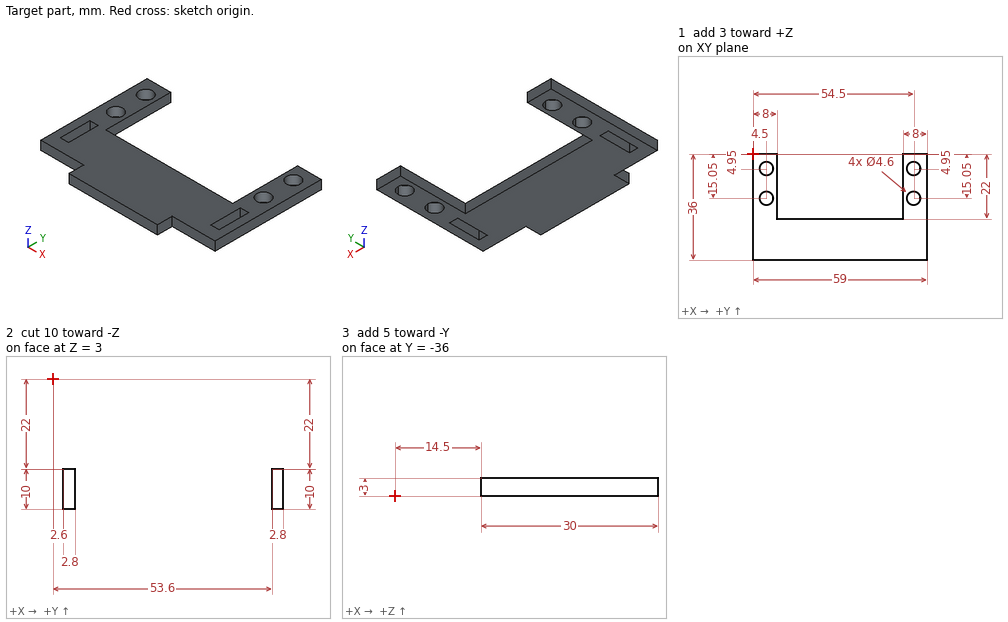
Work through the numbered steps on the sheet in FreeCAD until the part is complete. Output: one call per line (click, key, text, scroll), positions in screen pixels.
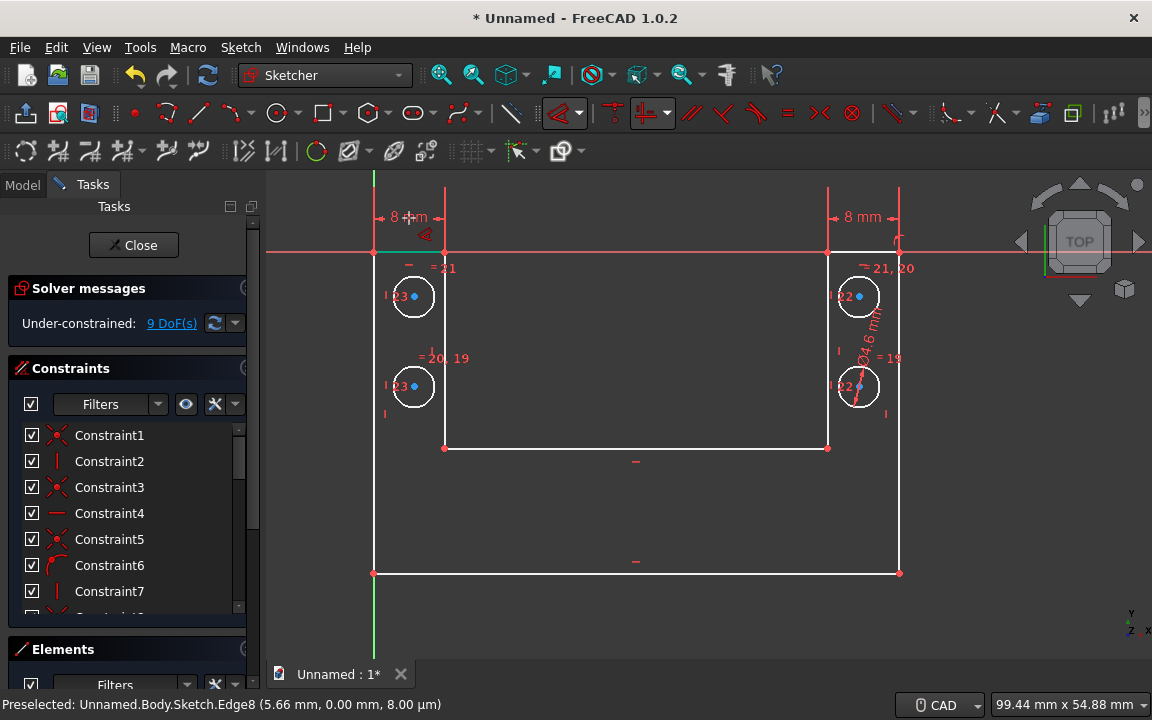
click(374, 349)
click(340, 413)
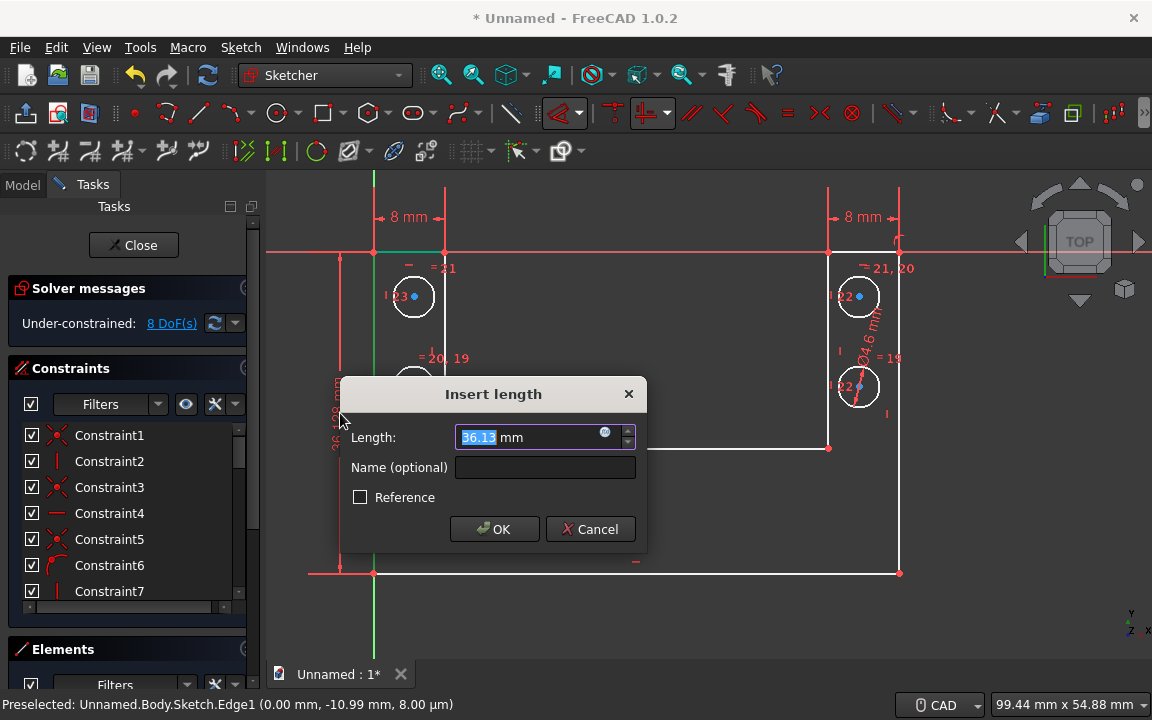
text(36)
key(Return)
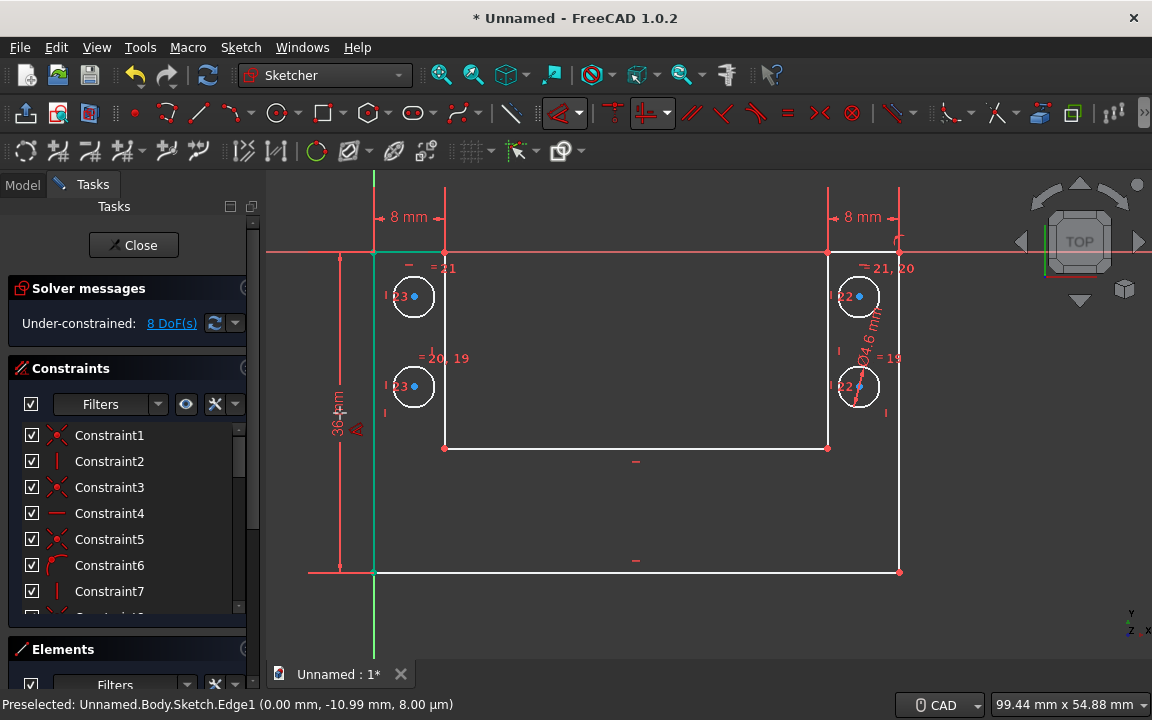
click(531, 573)
click(636, 607)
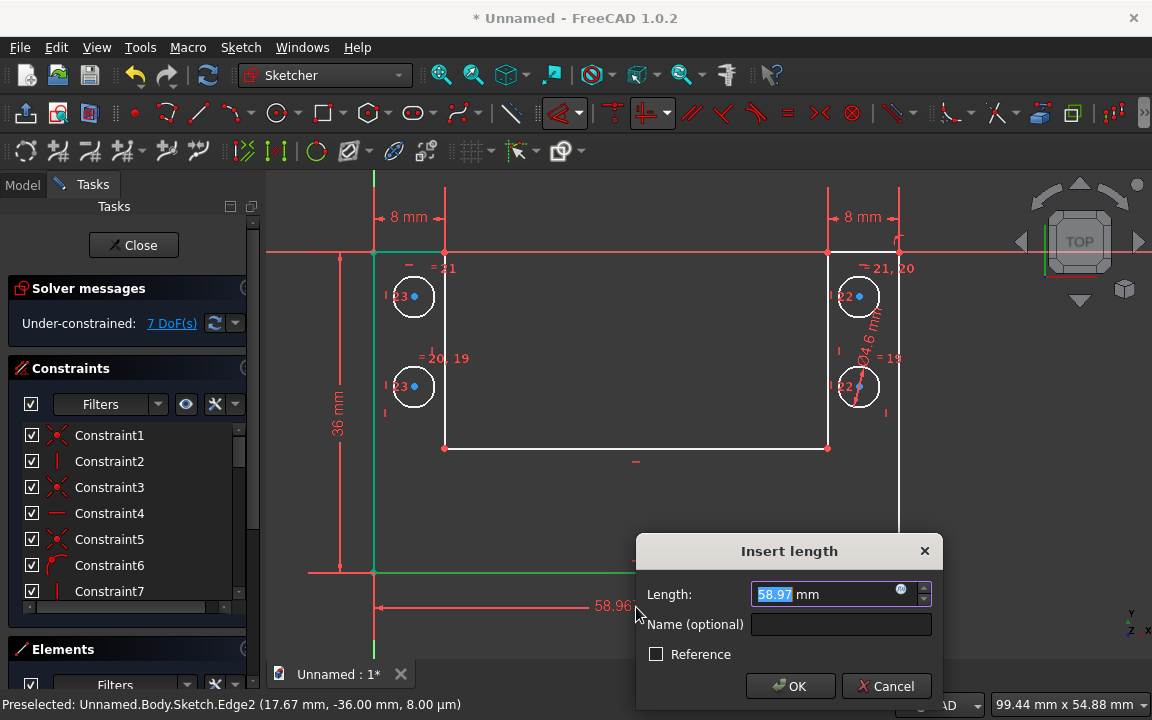
text(59)
key(Return)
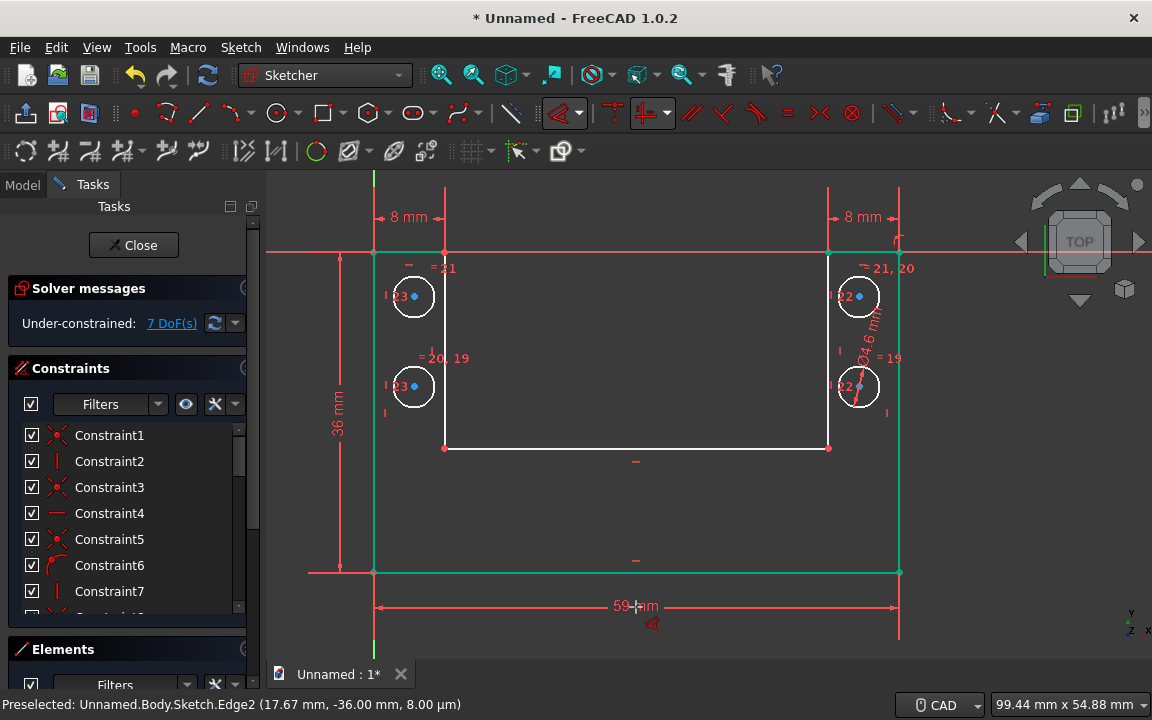
click(828, 311)
click(794, 351)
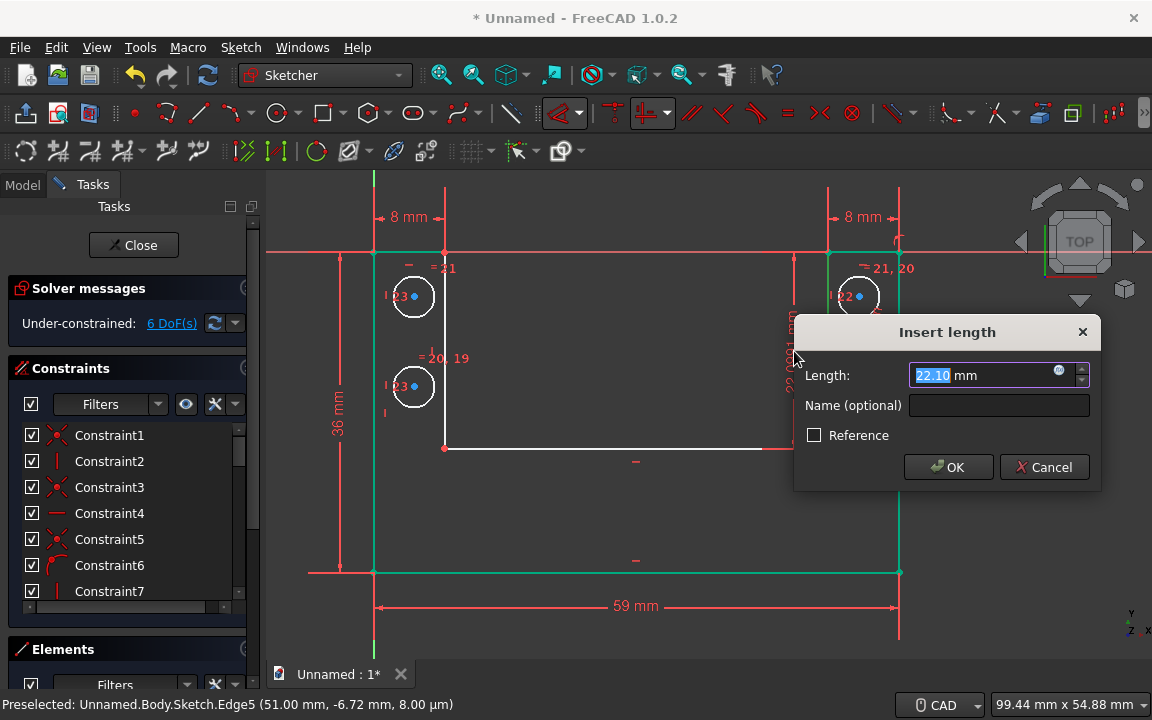
text(22)
key(Return)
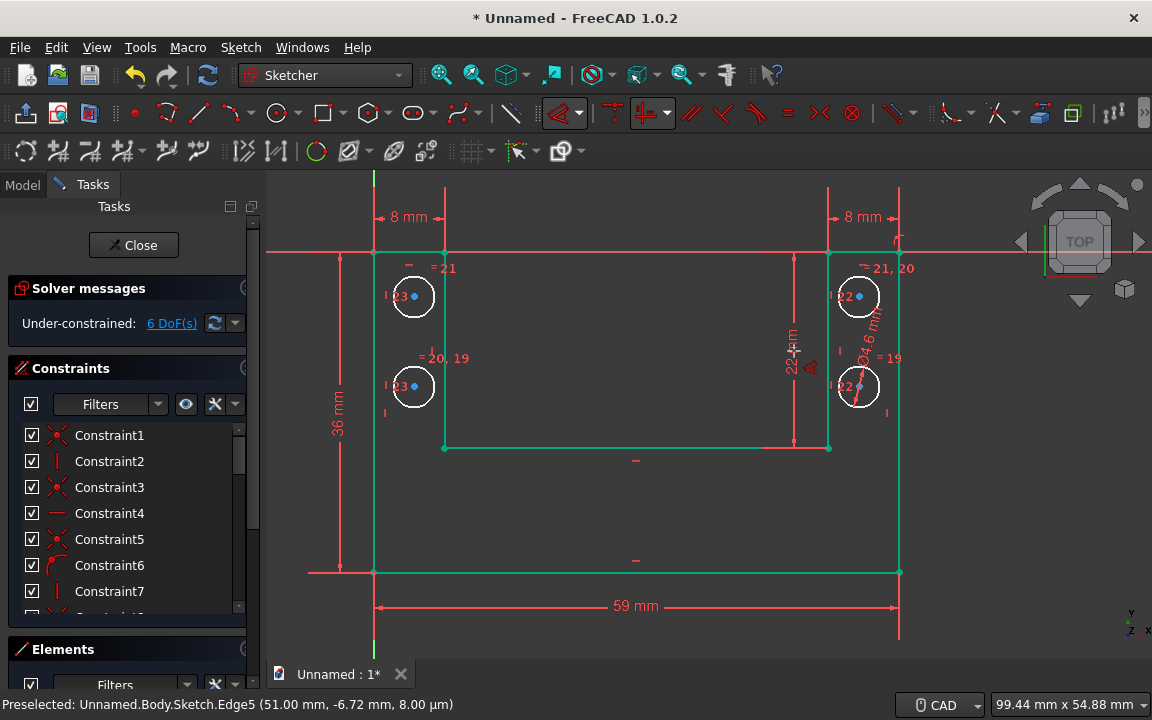
click(414, 387)
click(394, 445)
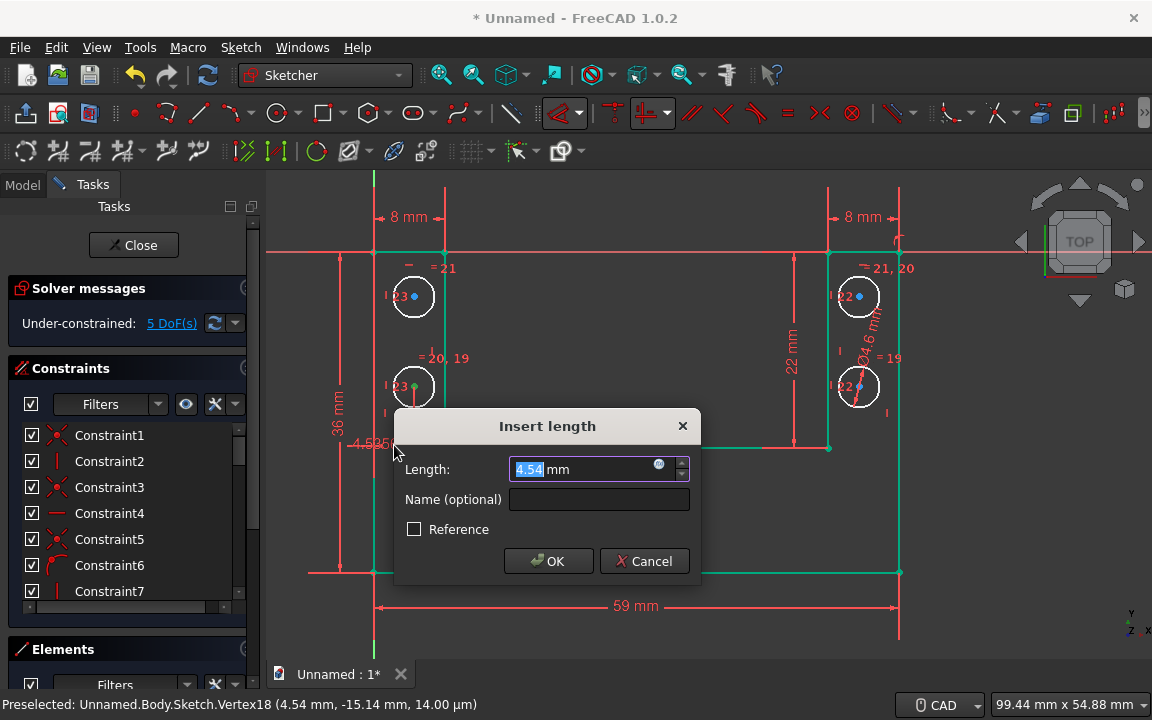
text(4.5)
key(Return)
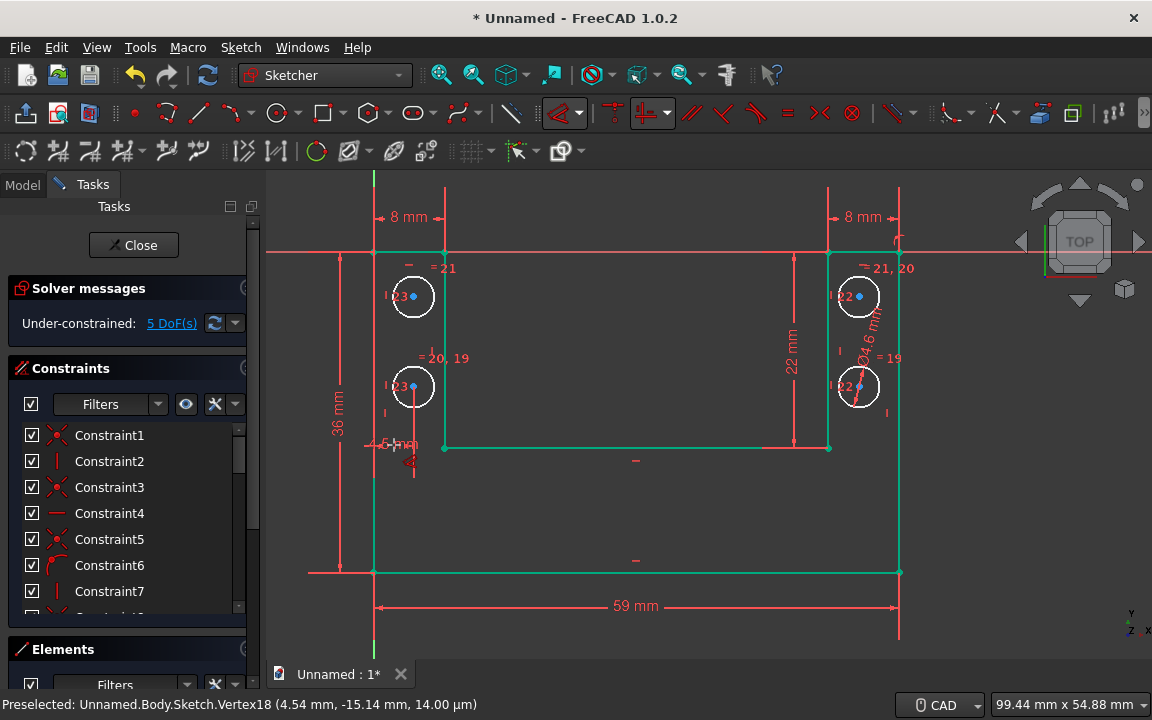
click(859, 387)
click(616, 218)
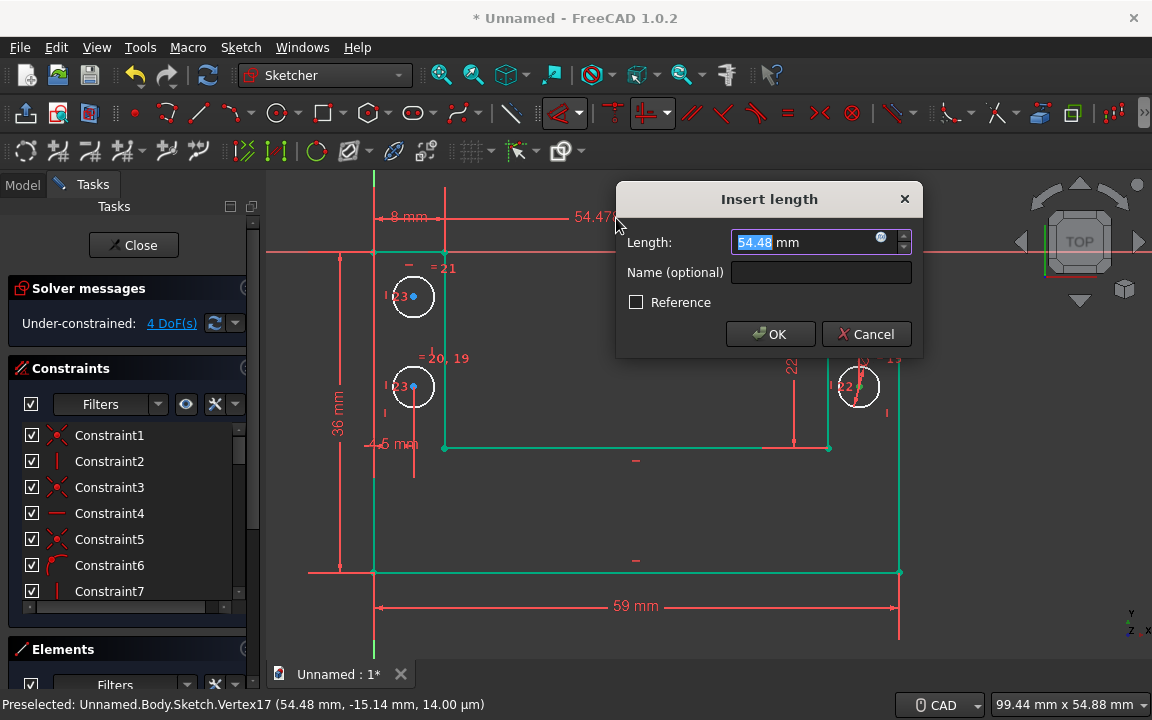
text(54.5)
key(Return)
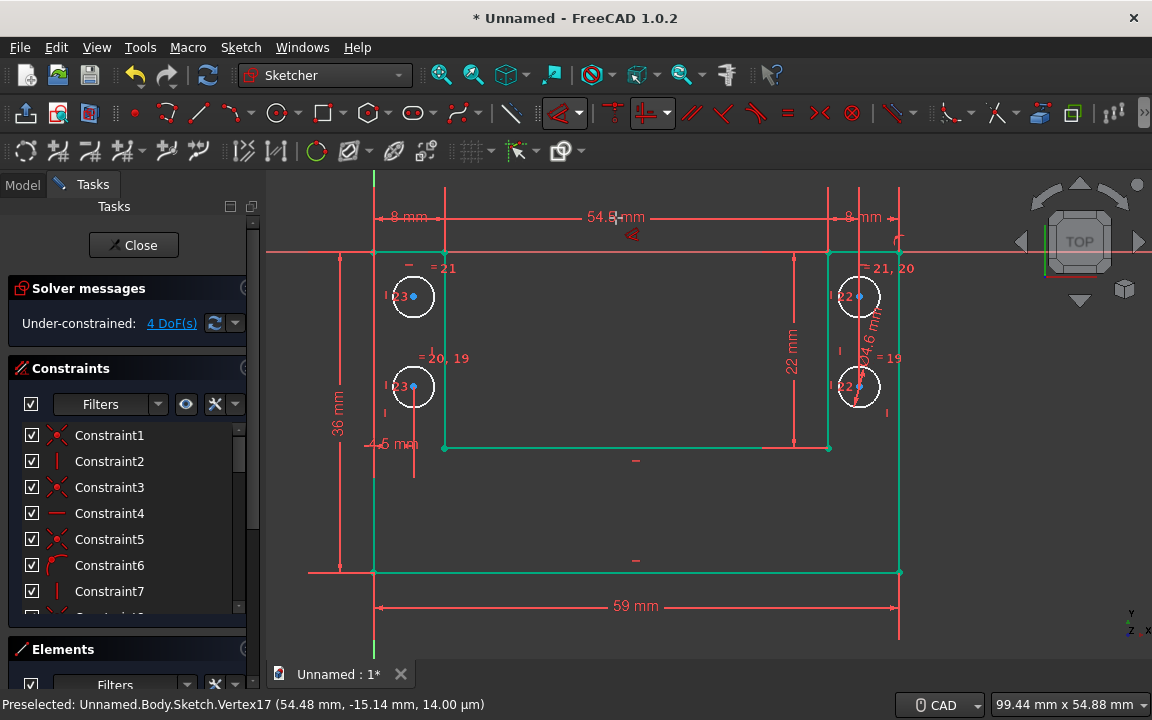
click(859, 297)
click(340, 275)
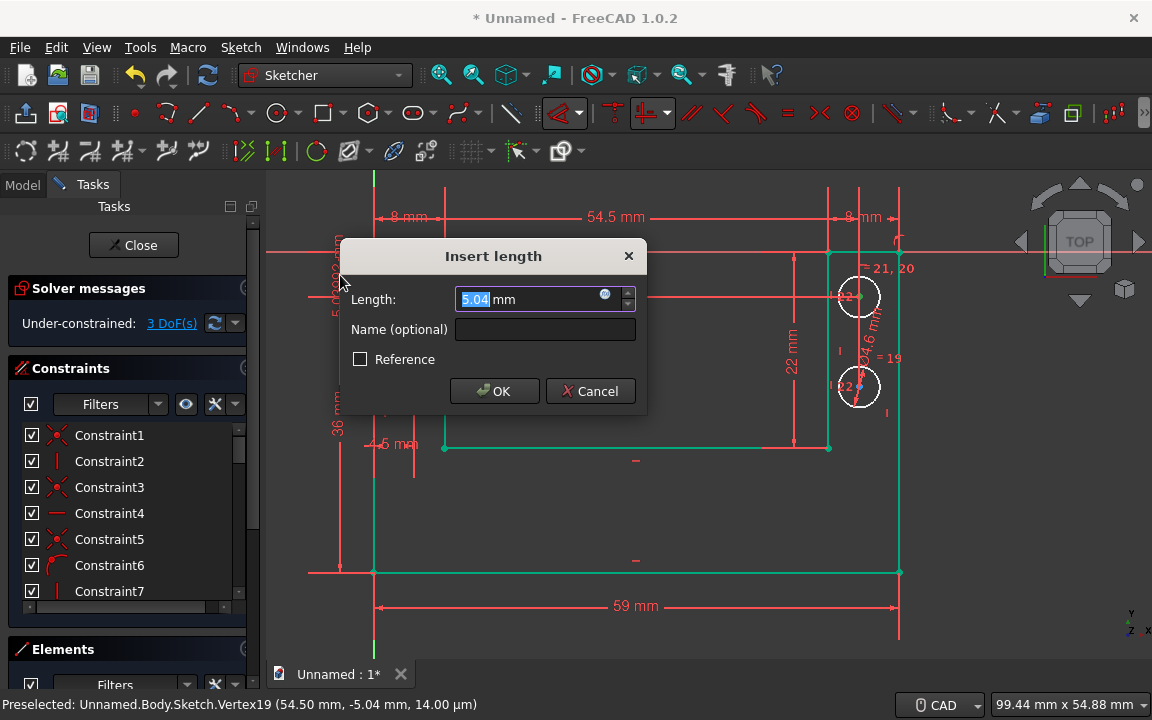
text(4.95)
key(Return)